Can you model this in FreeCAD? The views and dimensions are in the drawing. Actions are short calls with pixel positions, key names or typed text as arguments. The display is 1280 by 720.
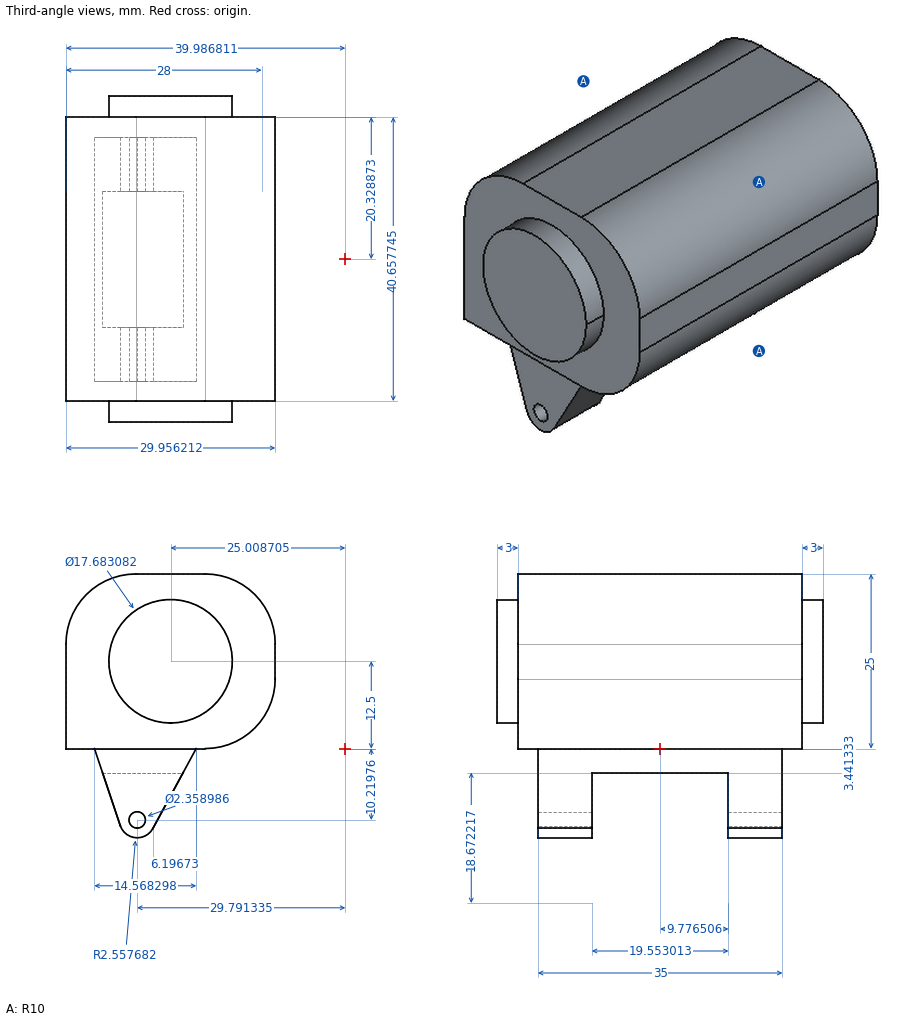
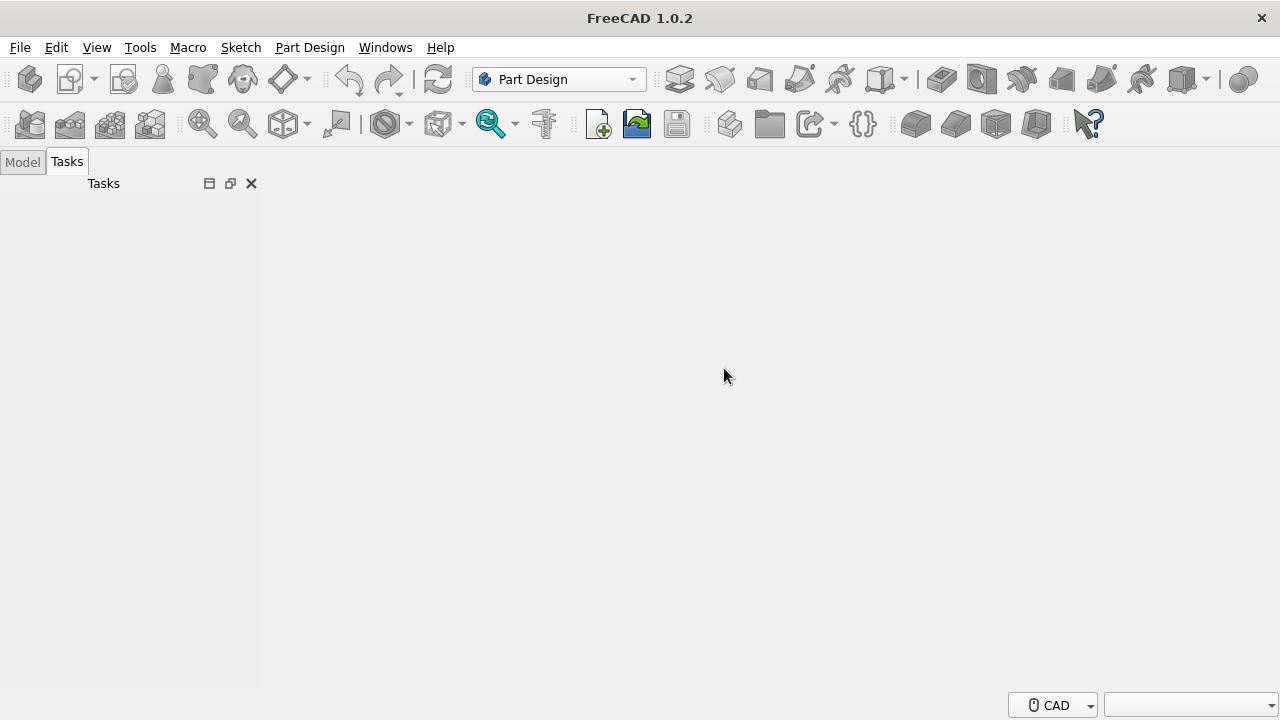
click(598, 124)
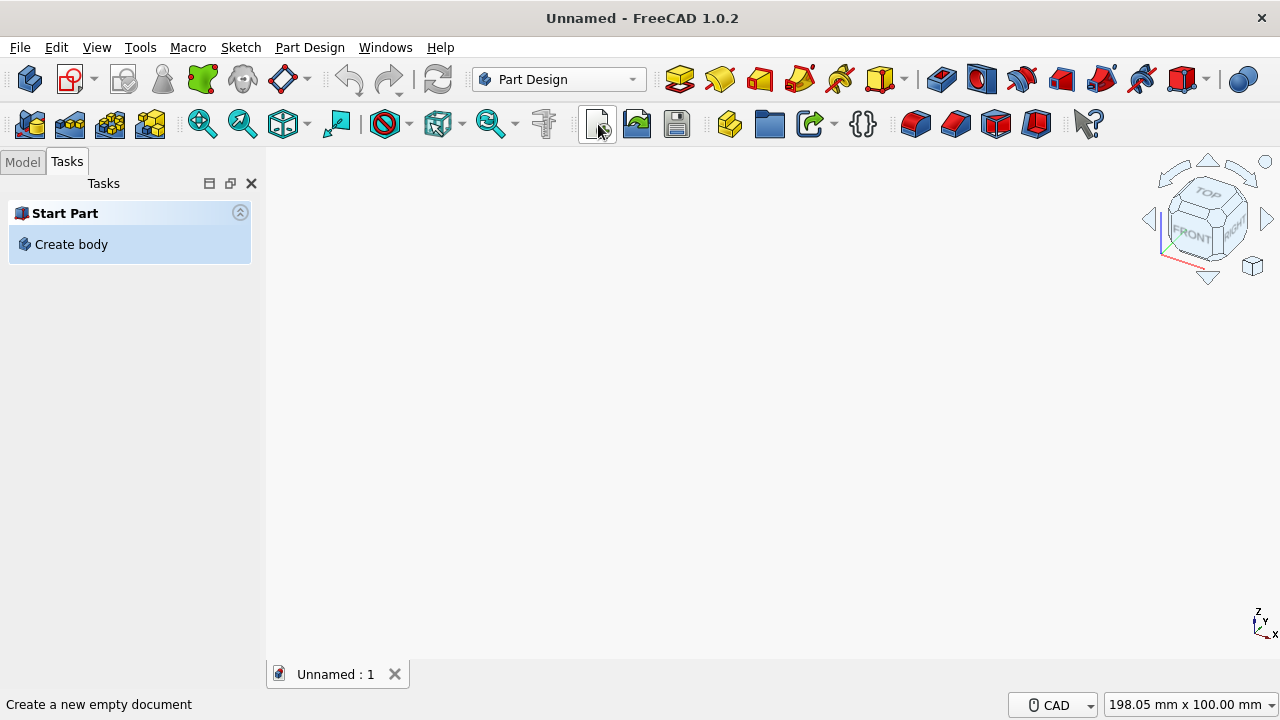
click(70, 80)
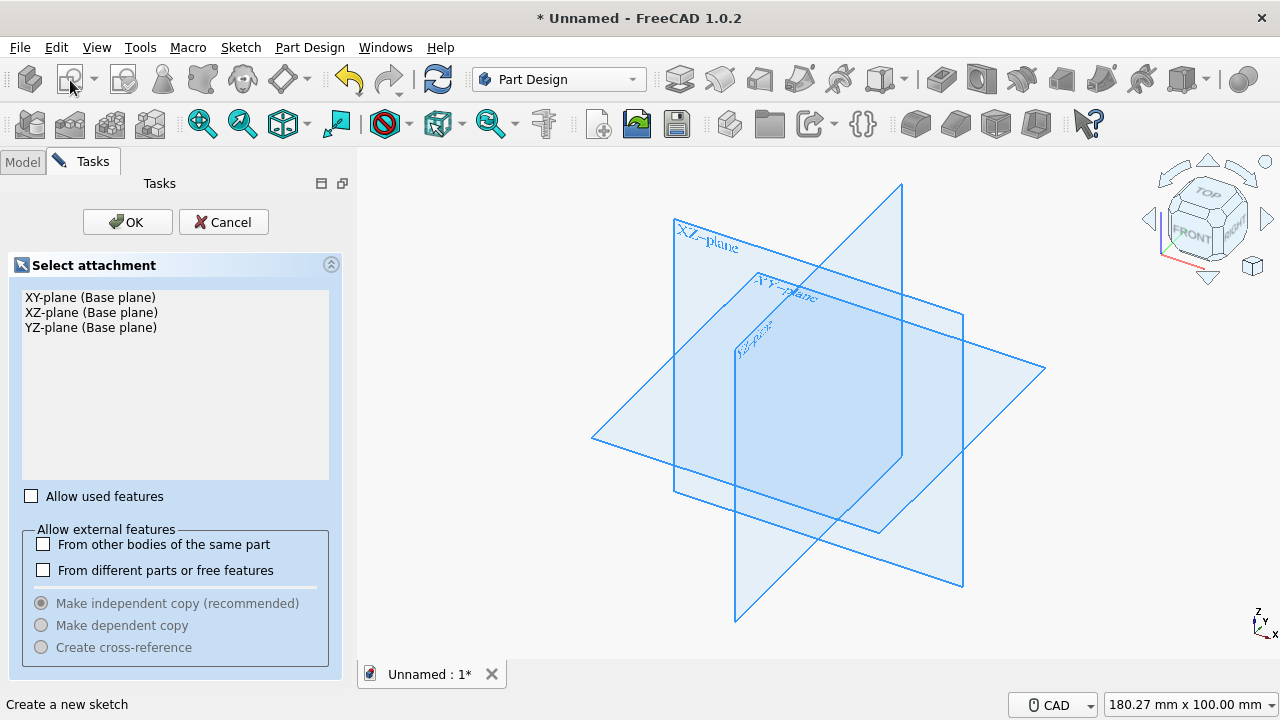
click(82, 298)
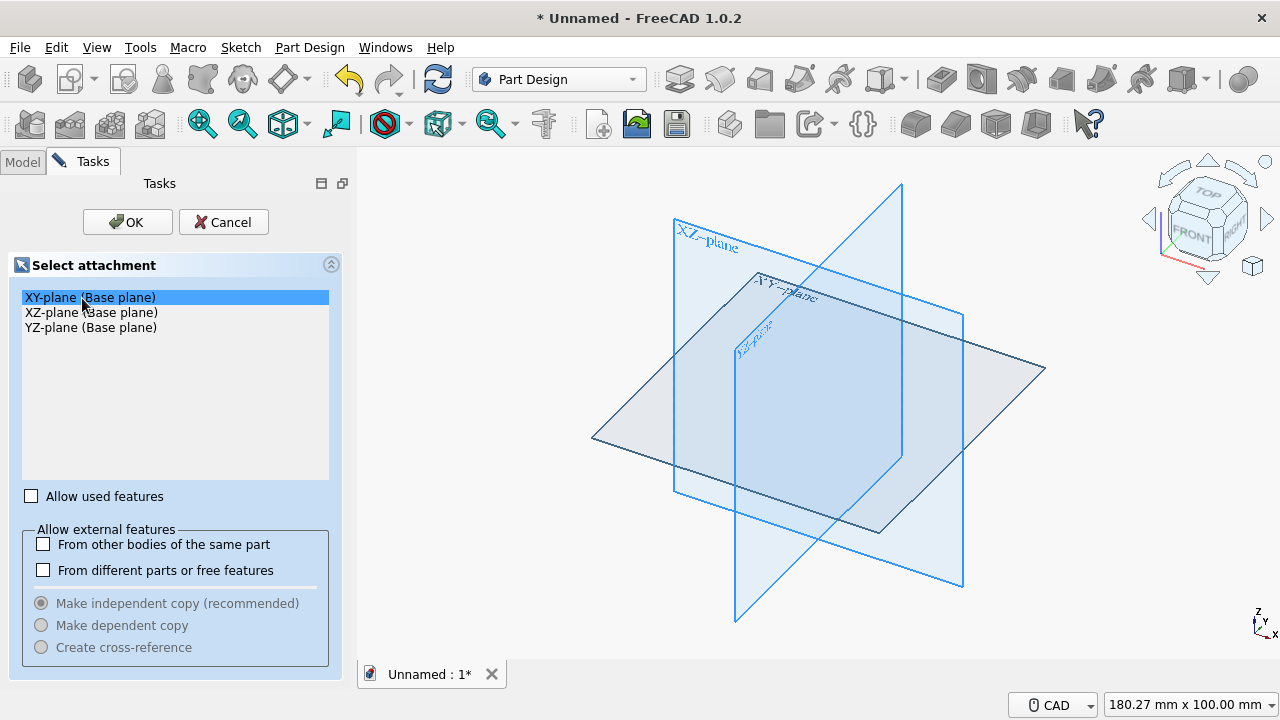
click(128, 222)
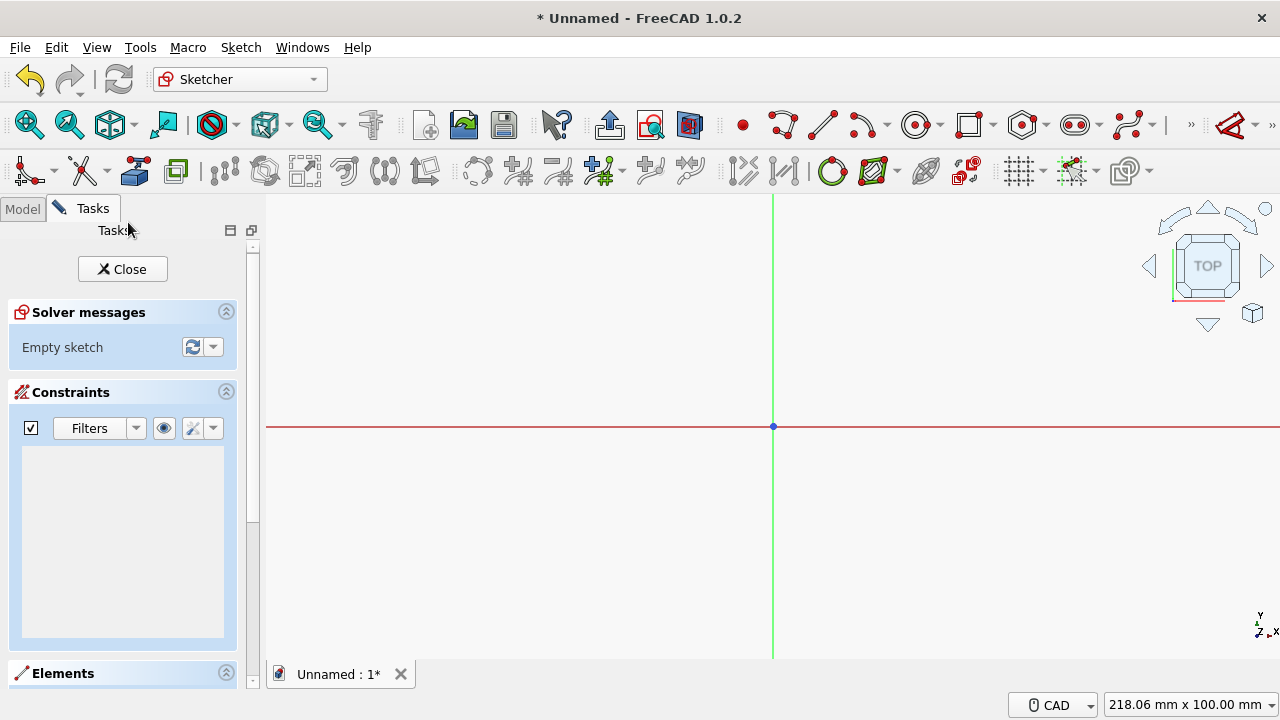
scroll(630, 426, up, 2)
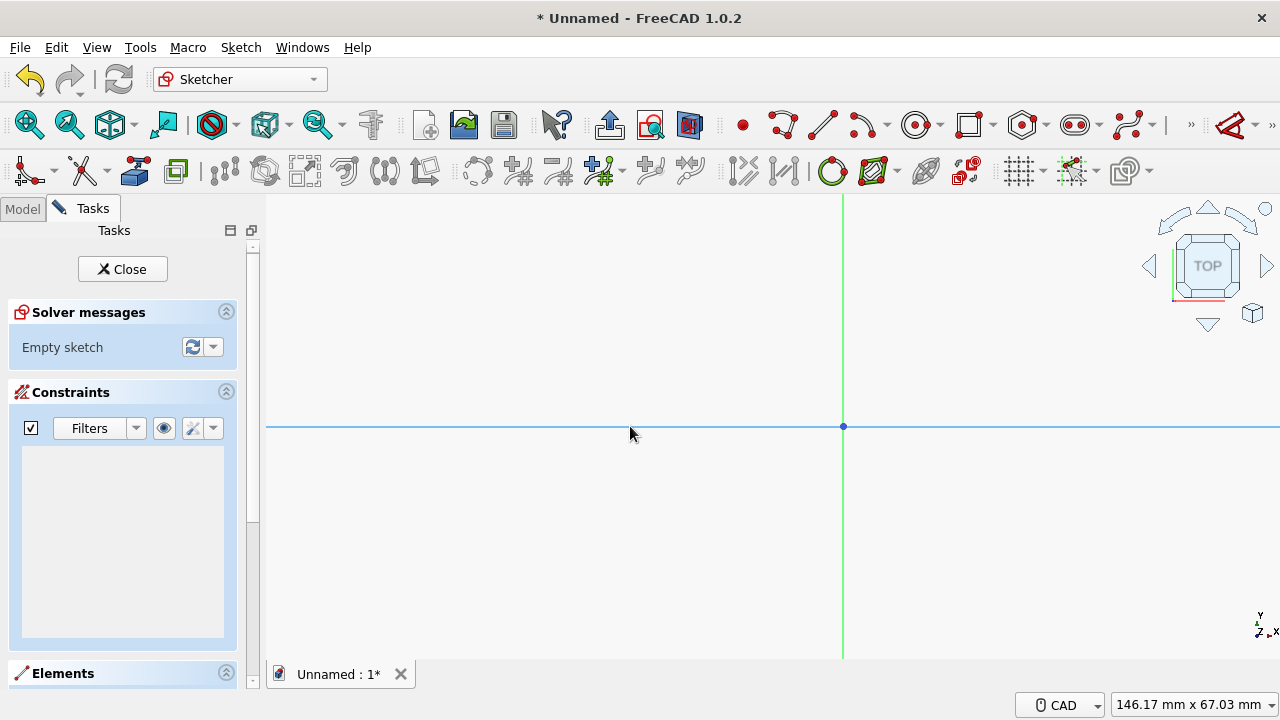
click(970, 126)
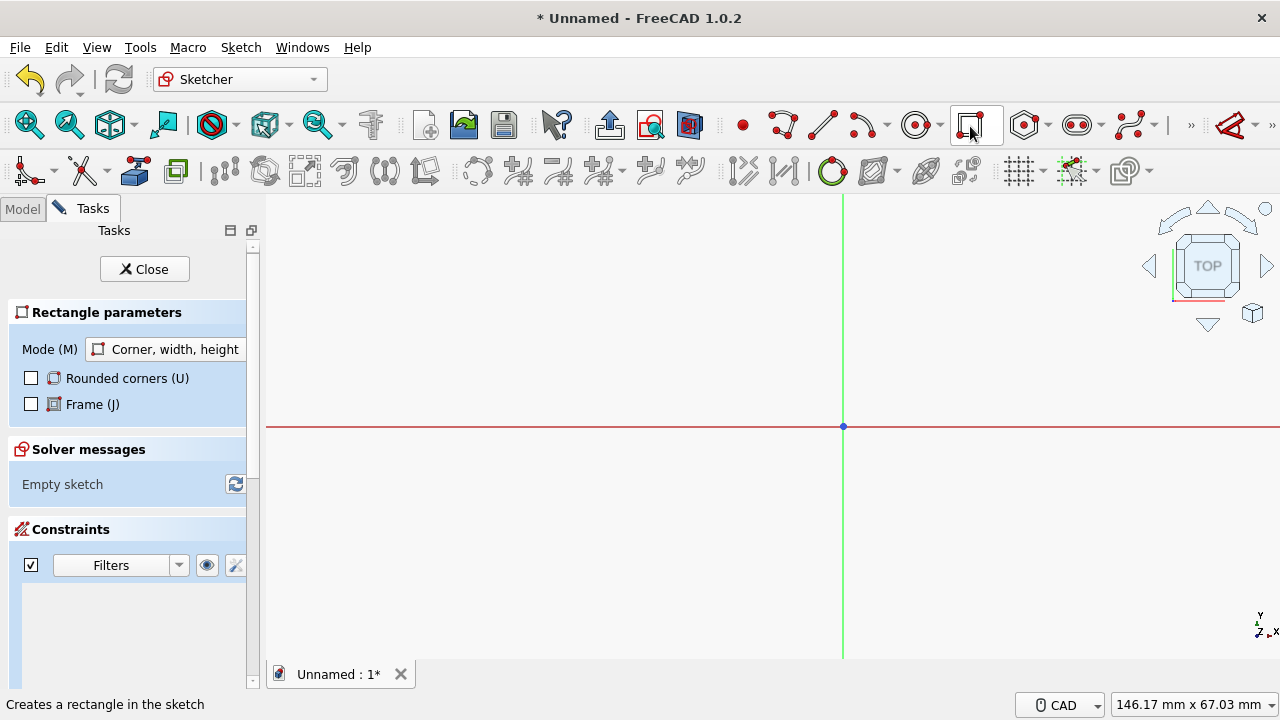
click(566, 285)
move(774, 568)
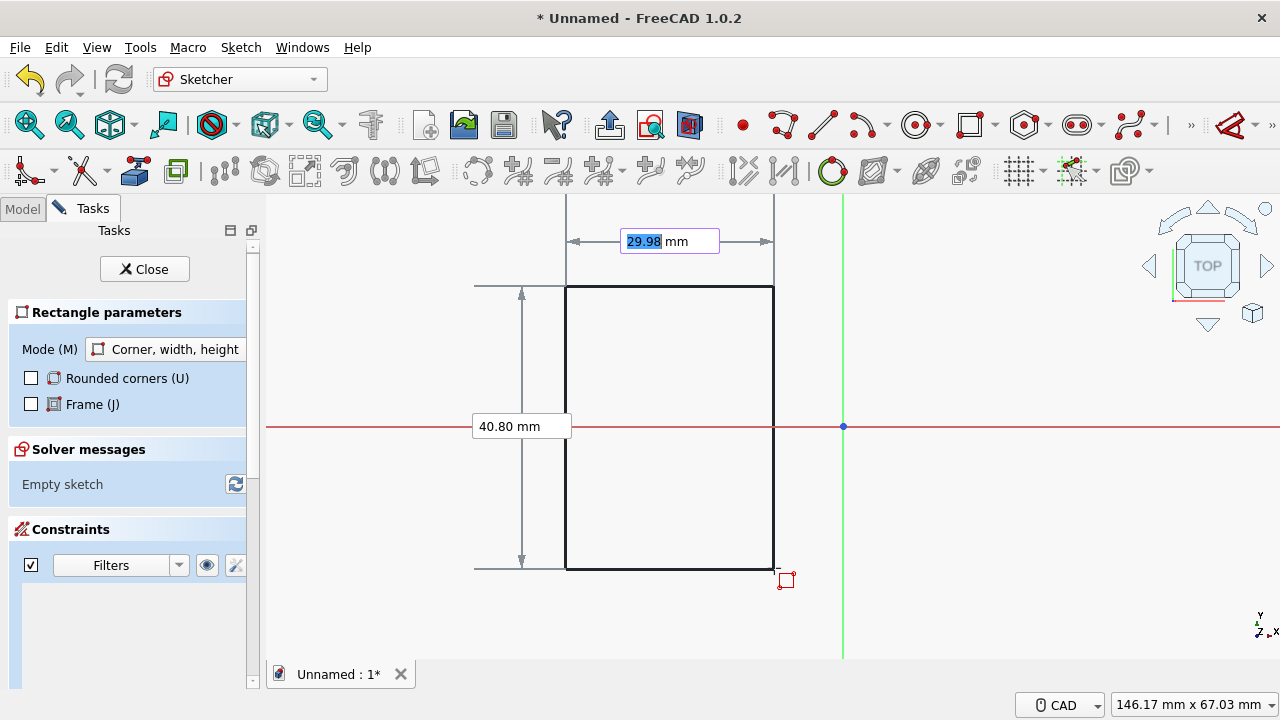
text(29.956212)
key(Tab)
text(40.657745)
key(Return)
key(Escape)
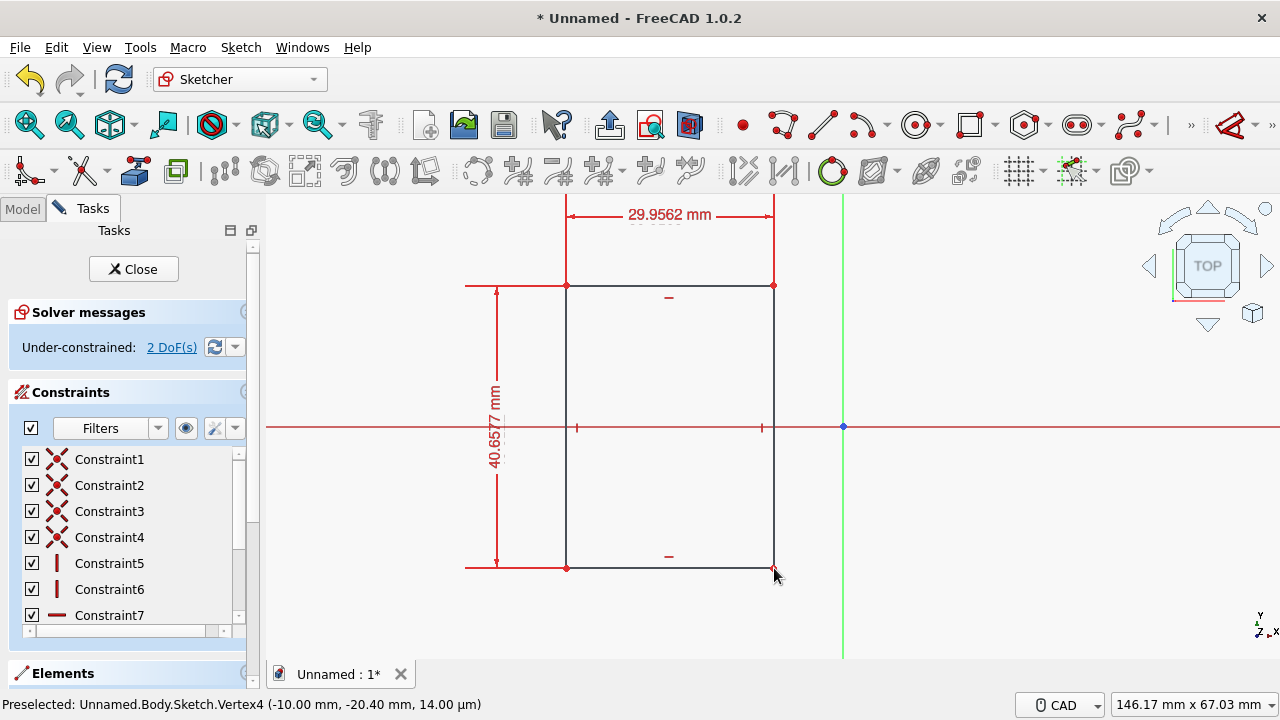
click(1230, 126)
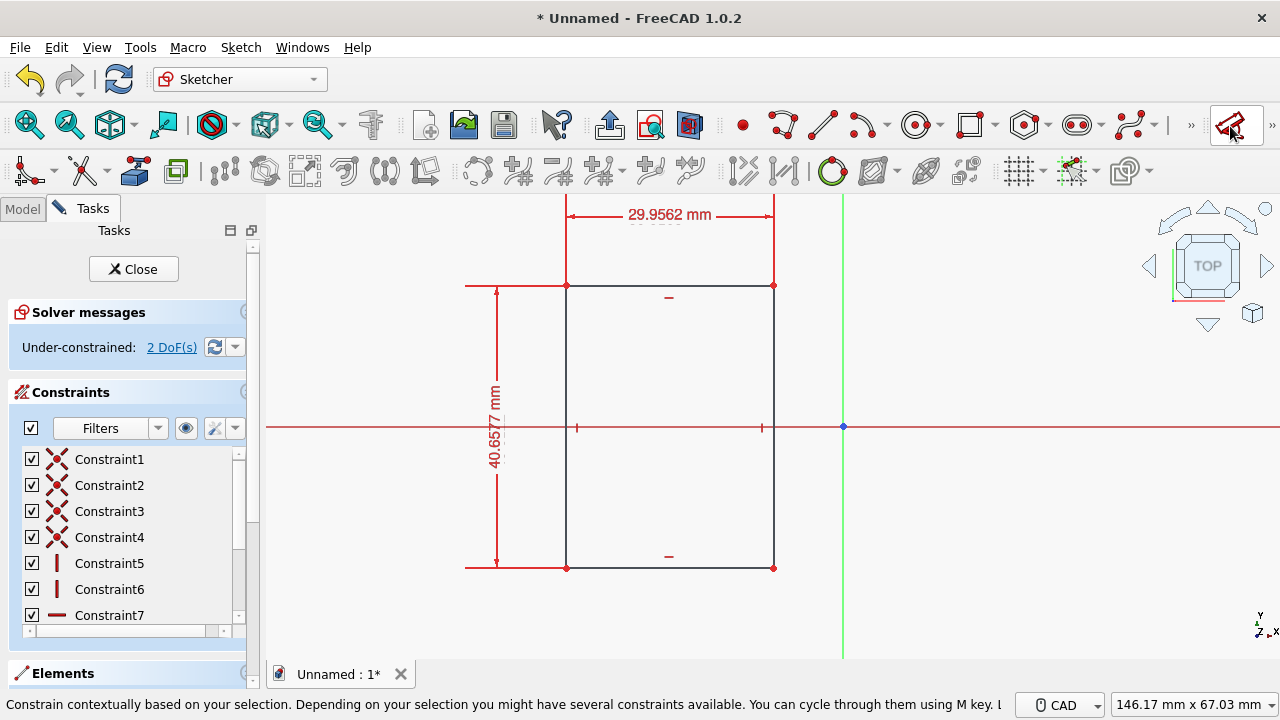
click(566, 286)
click(705, 252)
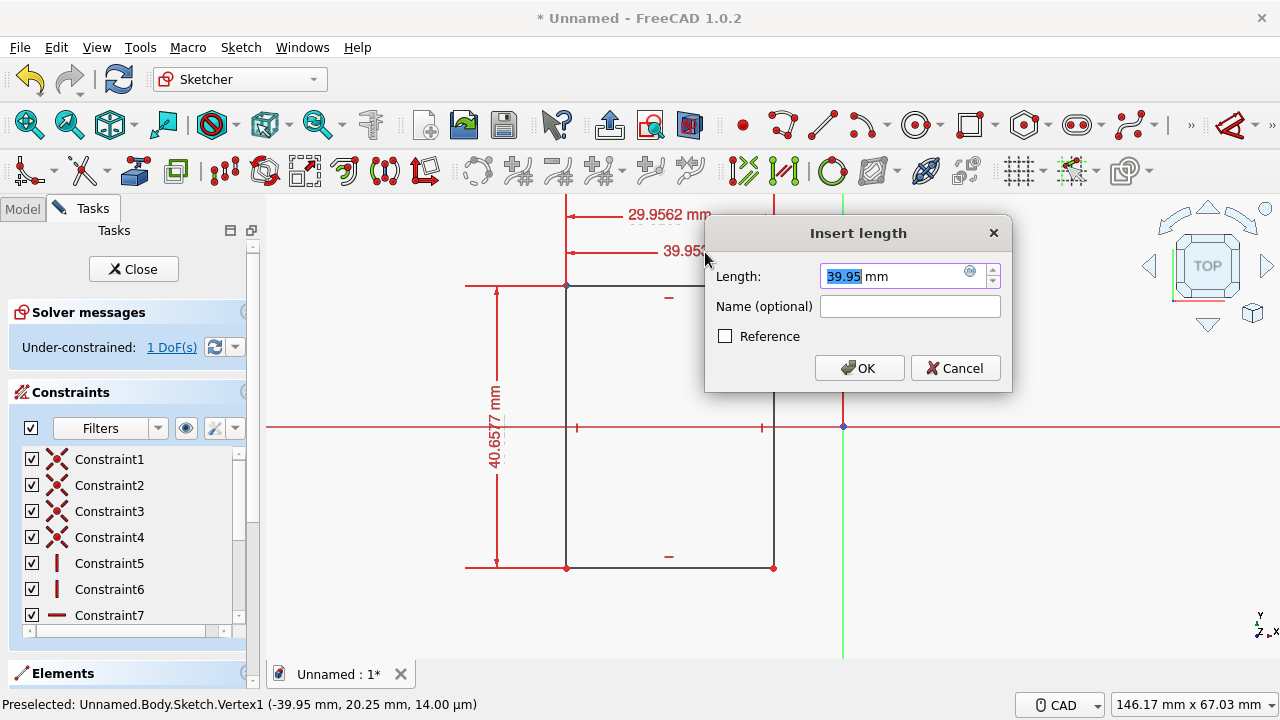
text(39.986811)
key(Return)